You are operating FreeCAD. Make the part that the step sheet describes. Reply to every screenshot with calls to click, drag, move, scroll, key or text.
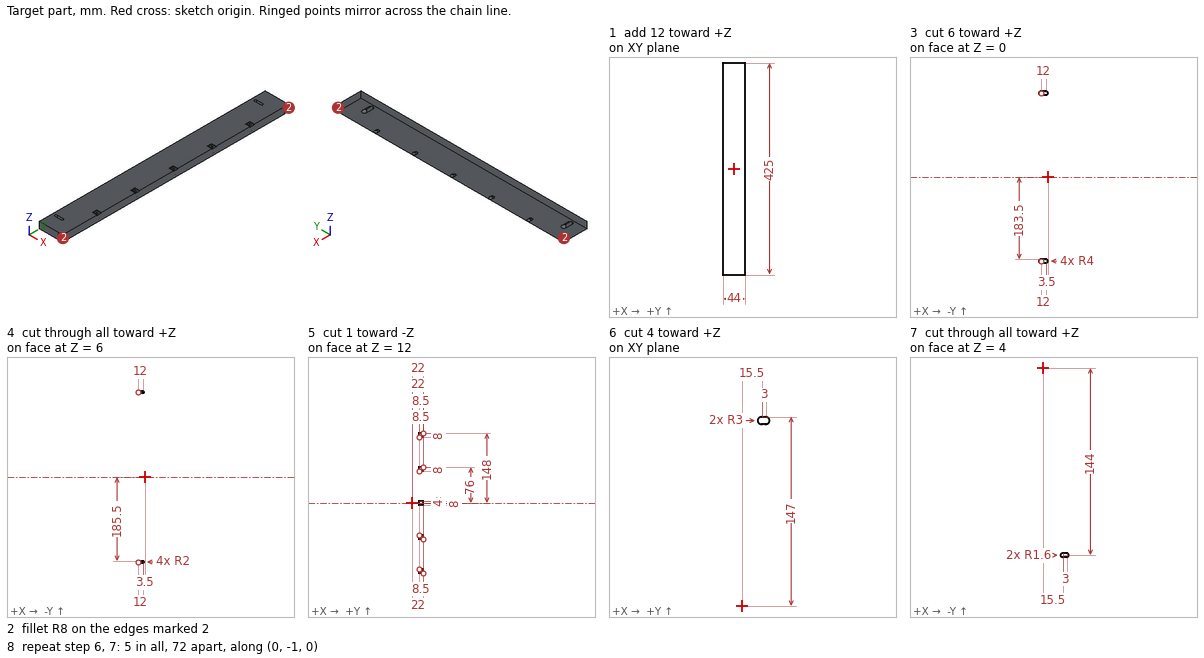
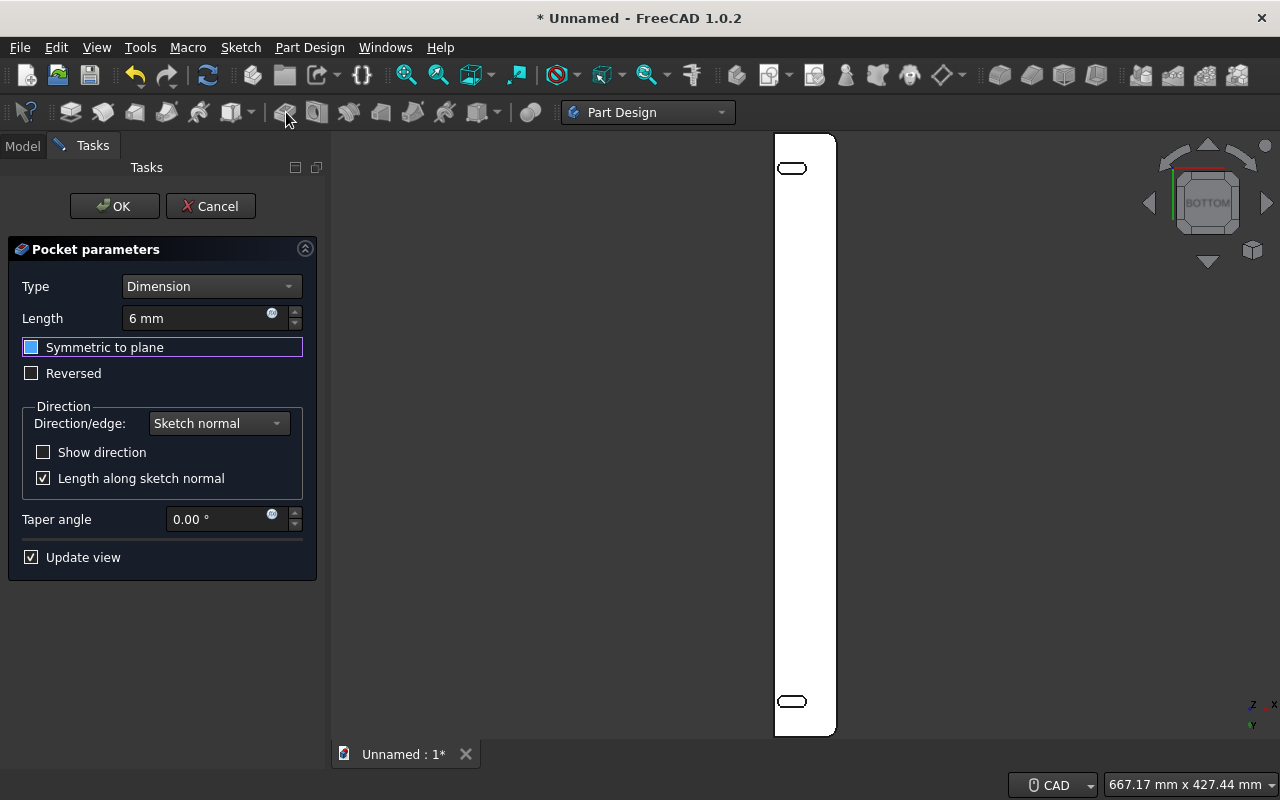
click(115, 206)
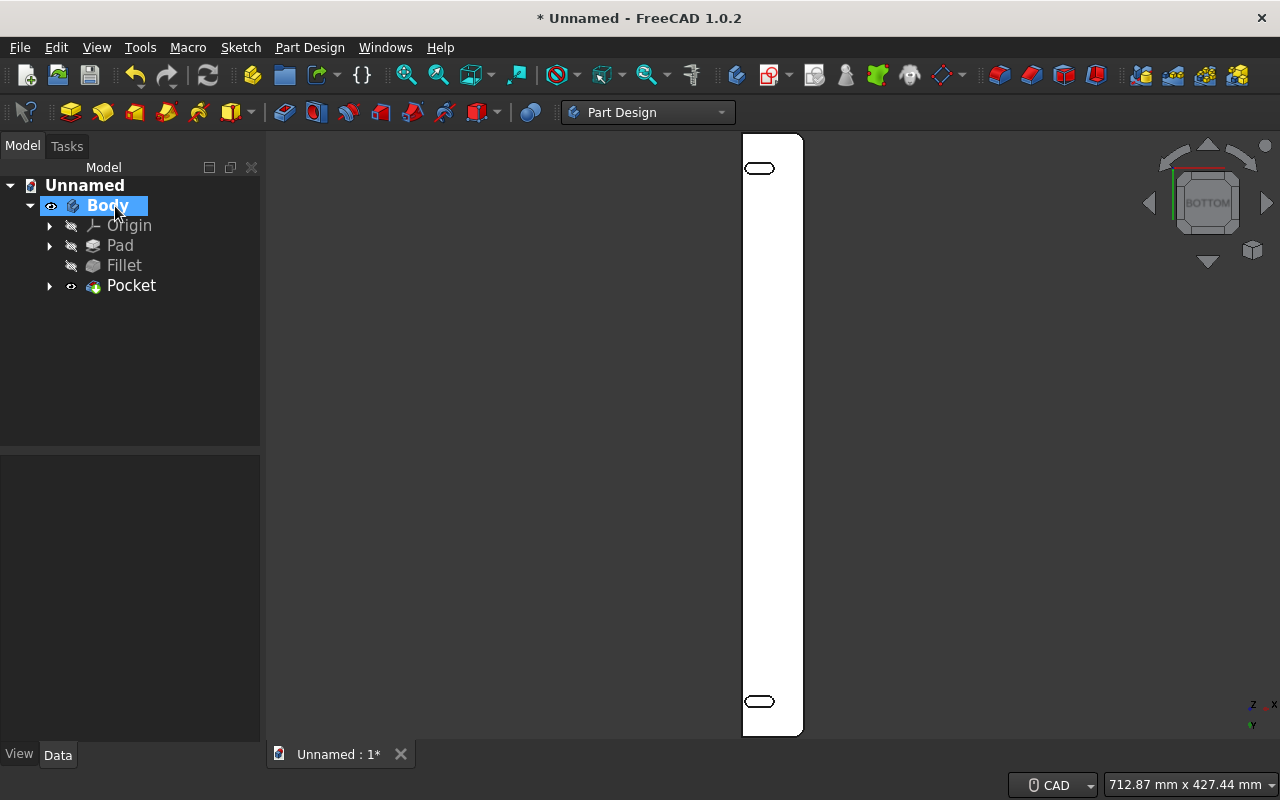
scroll(768, 701, up, 4)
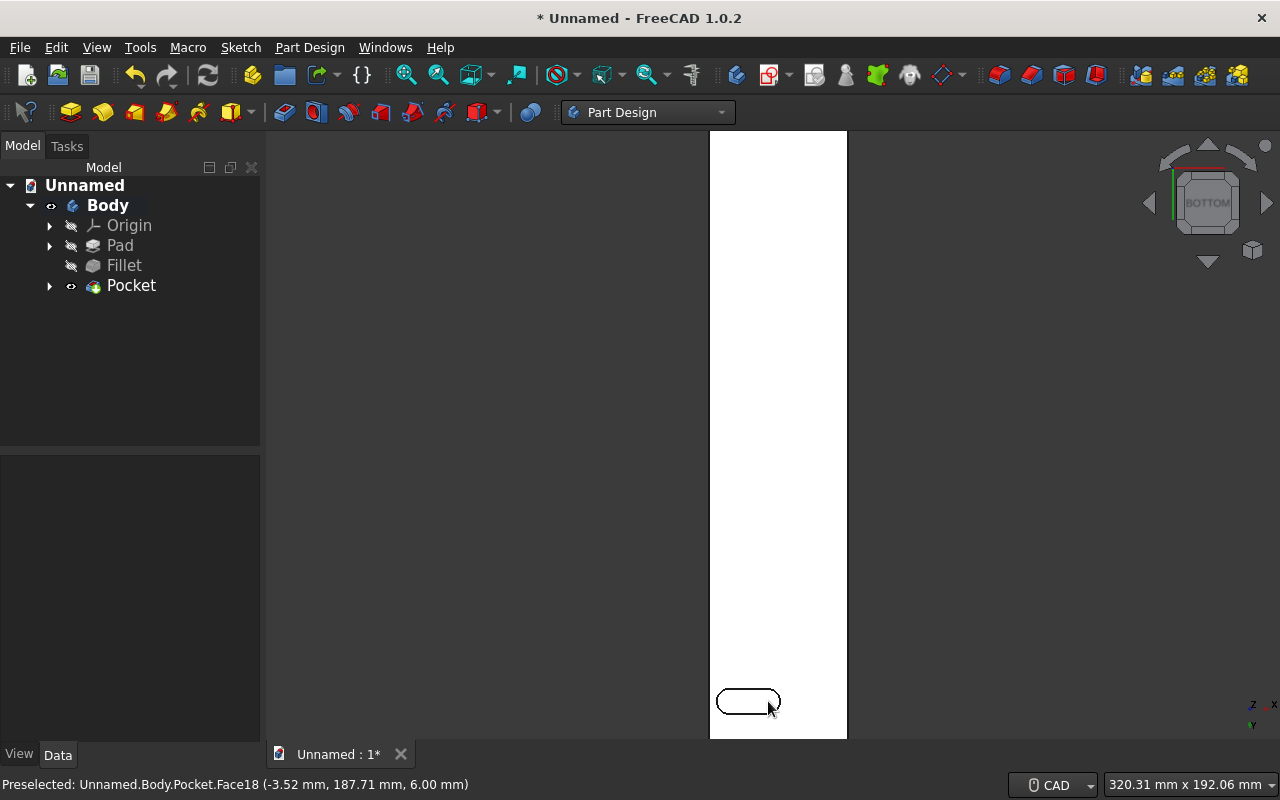
click(767, 700)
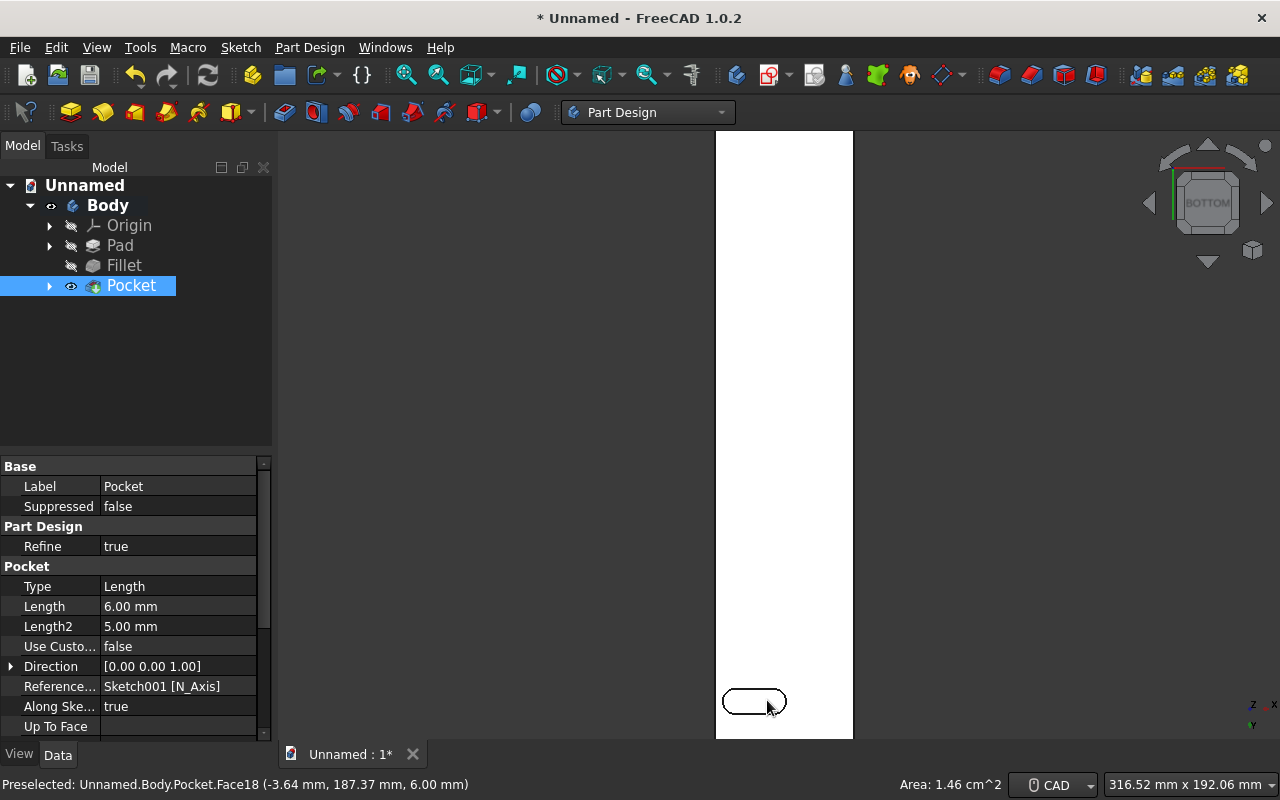
click(770, 76)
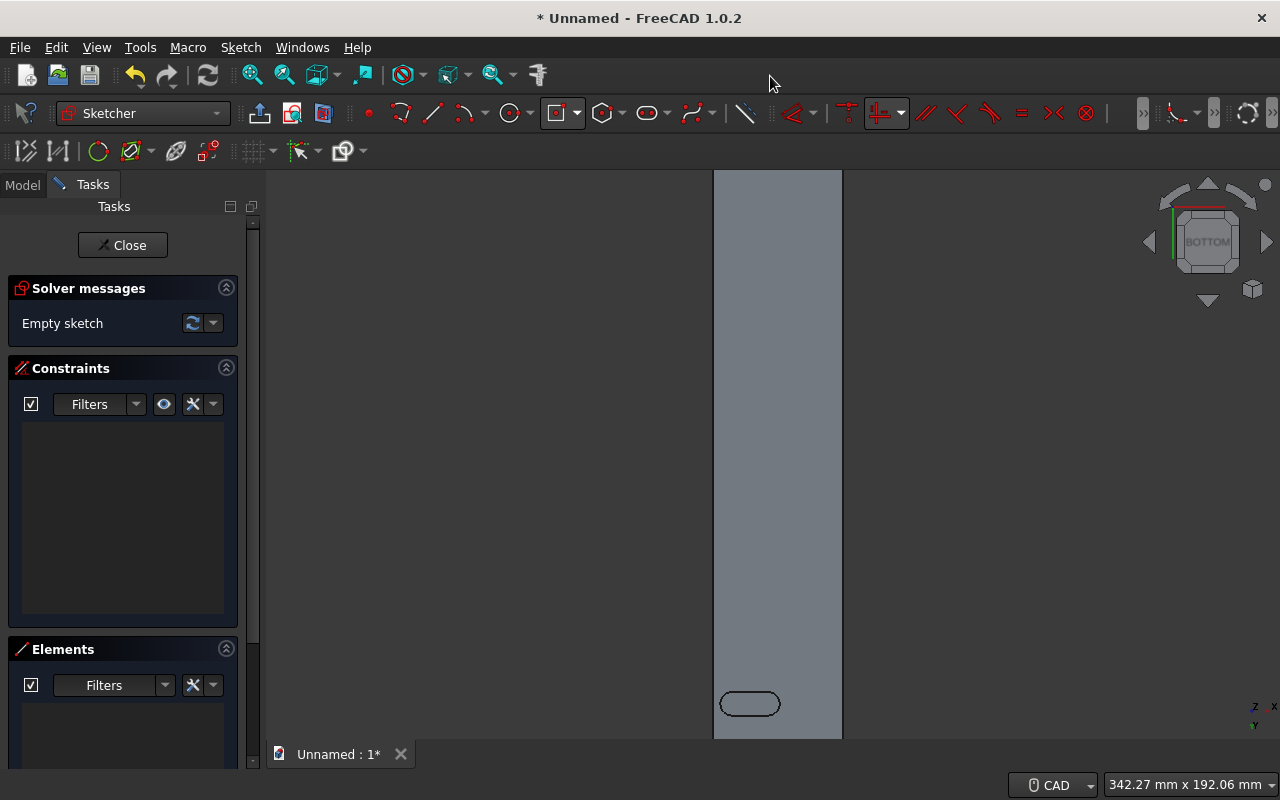
scroll(684, 586, down, 6)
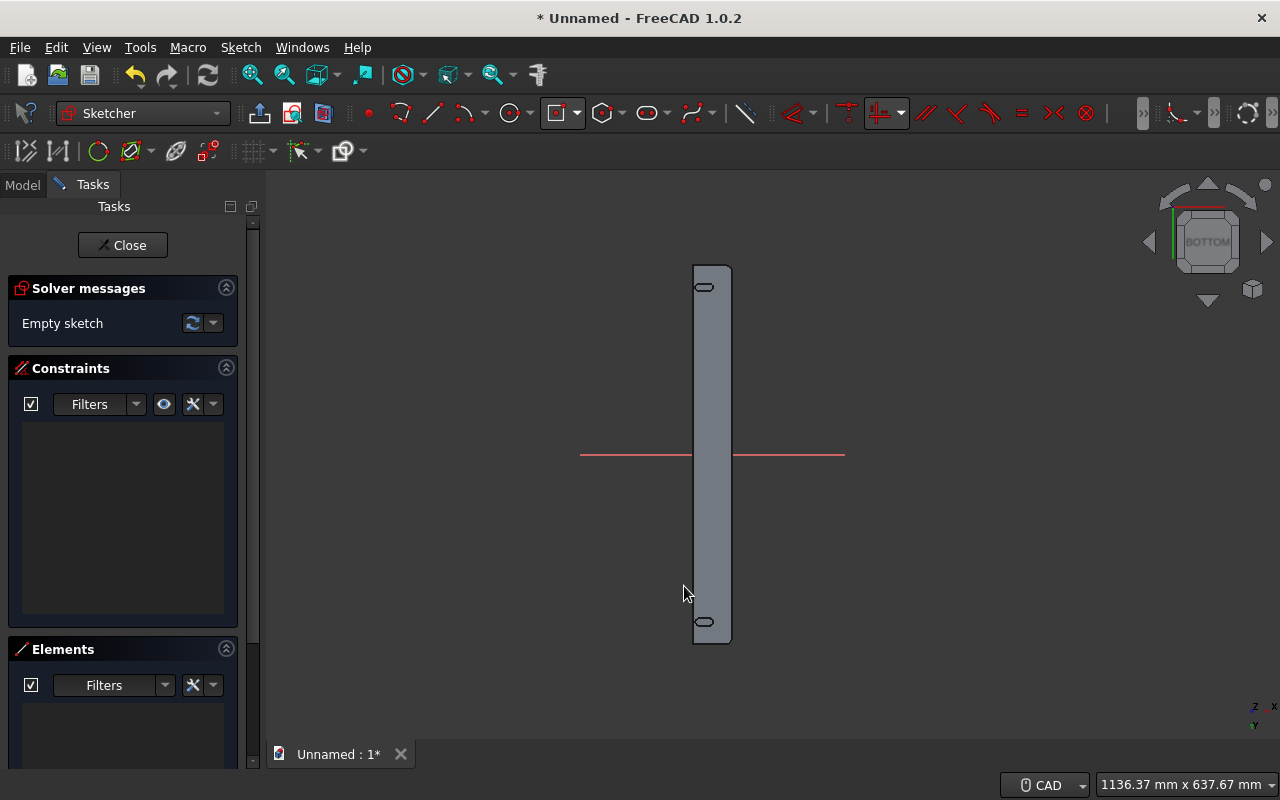
click(648, 114)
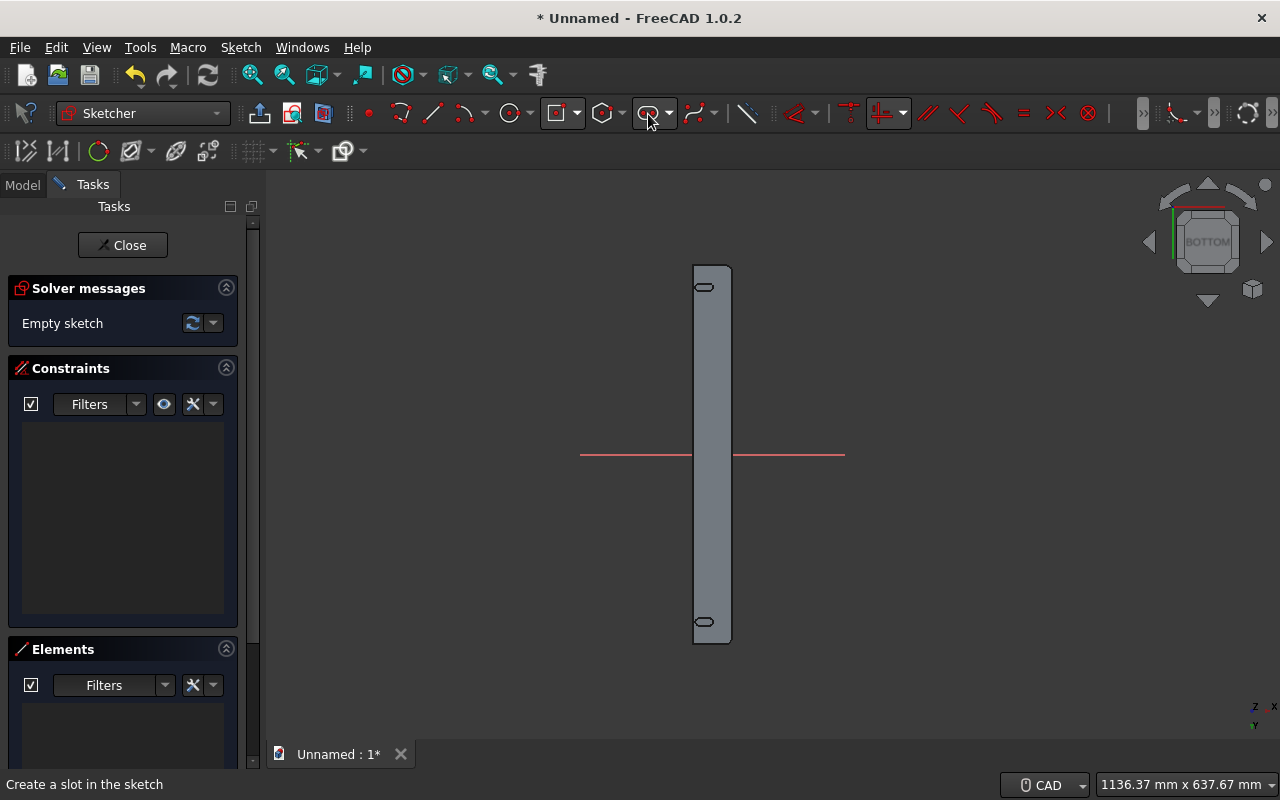
scroll(699, 622, up, 13)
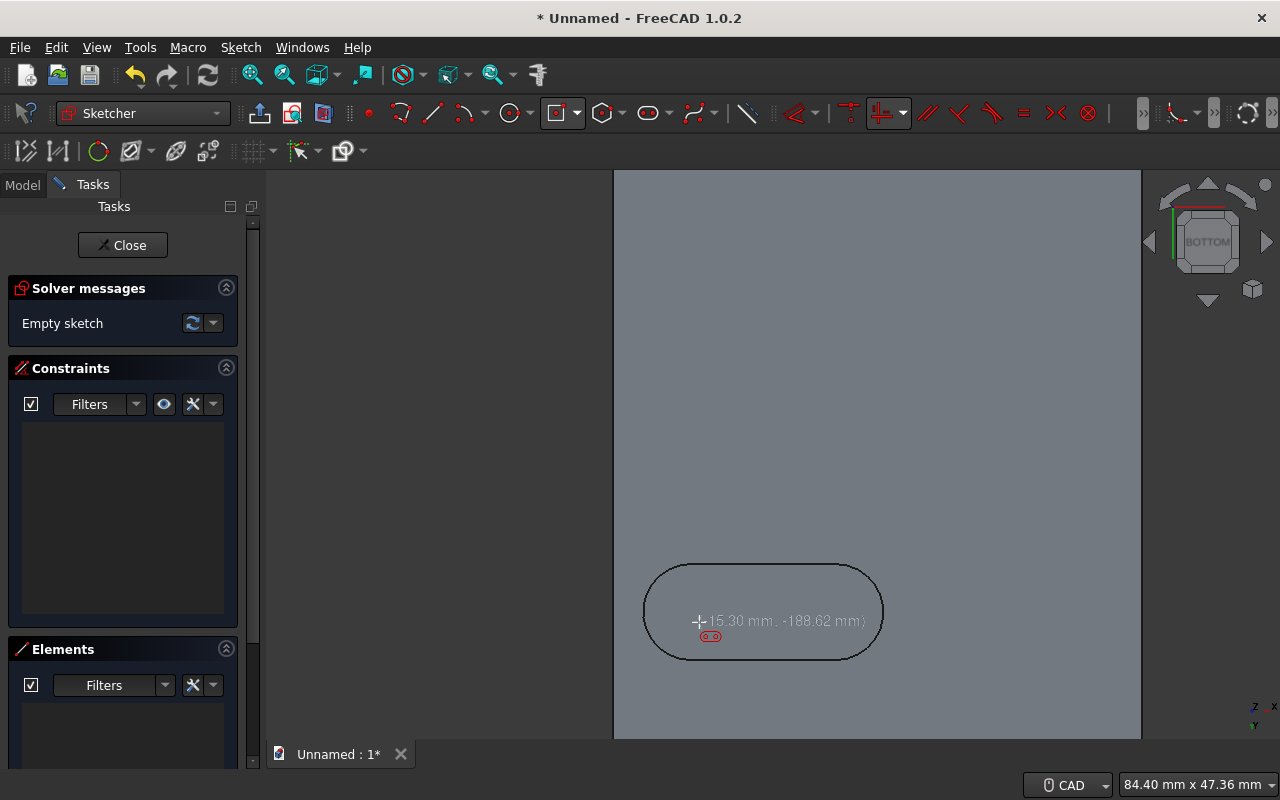
scroll(699, 623, down, 13)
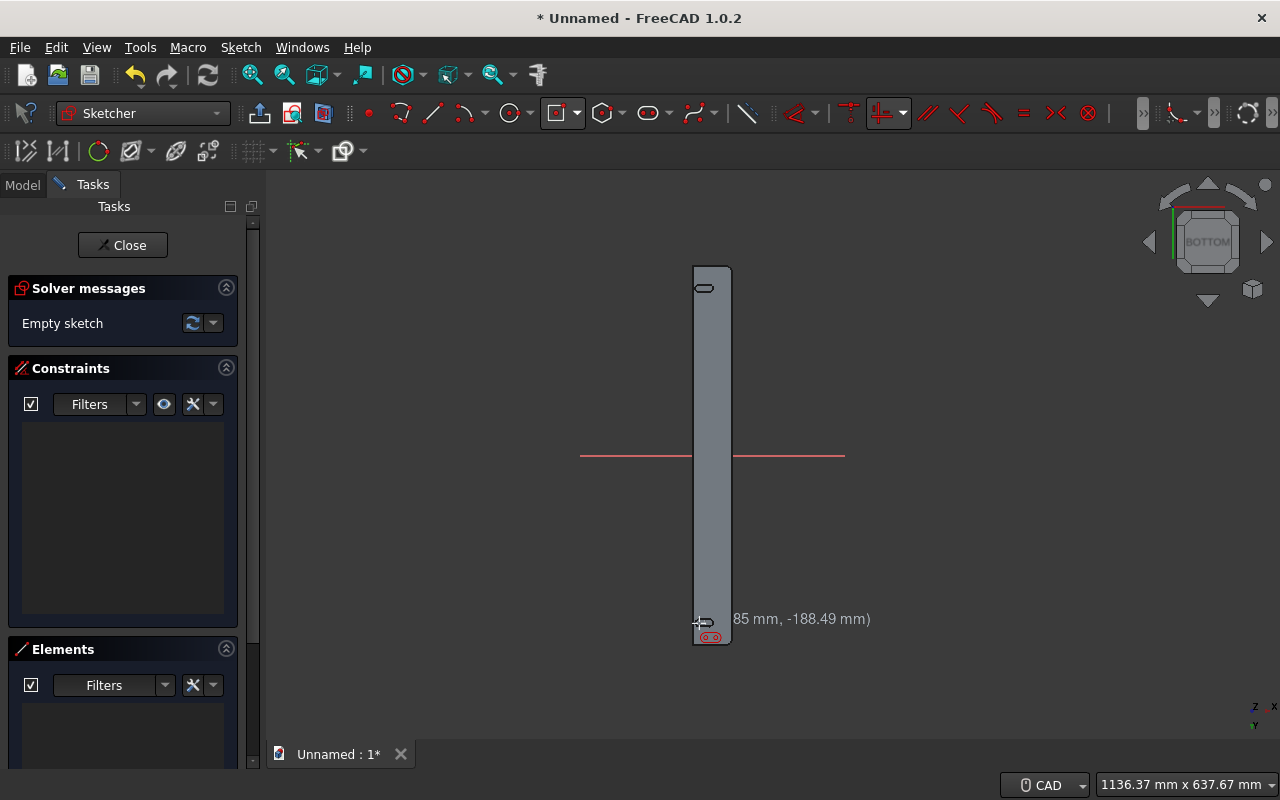
click(699, 623)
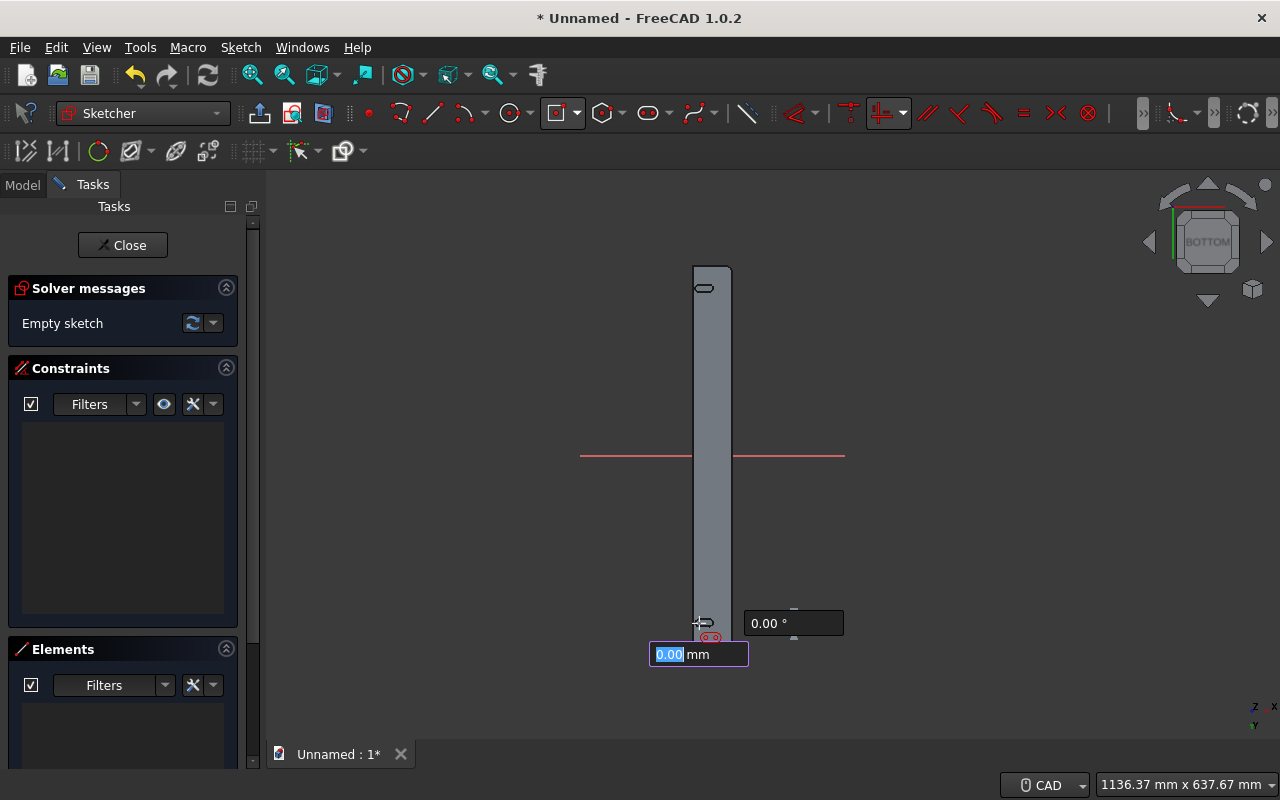
scroll(710, 623, up, 9)